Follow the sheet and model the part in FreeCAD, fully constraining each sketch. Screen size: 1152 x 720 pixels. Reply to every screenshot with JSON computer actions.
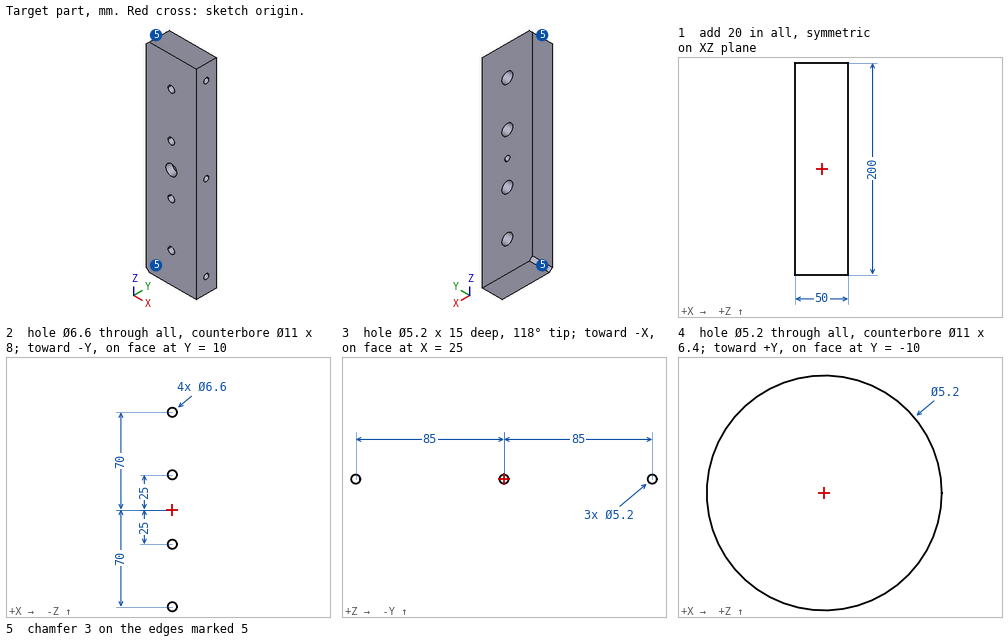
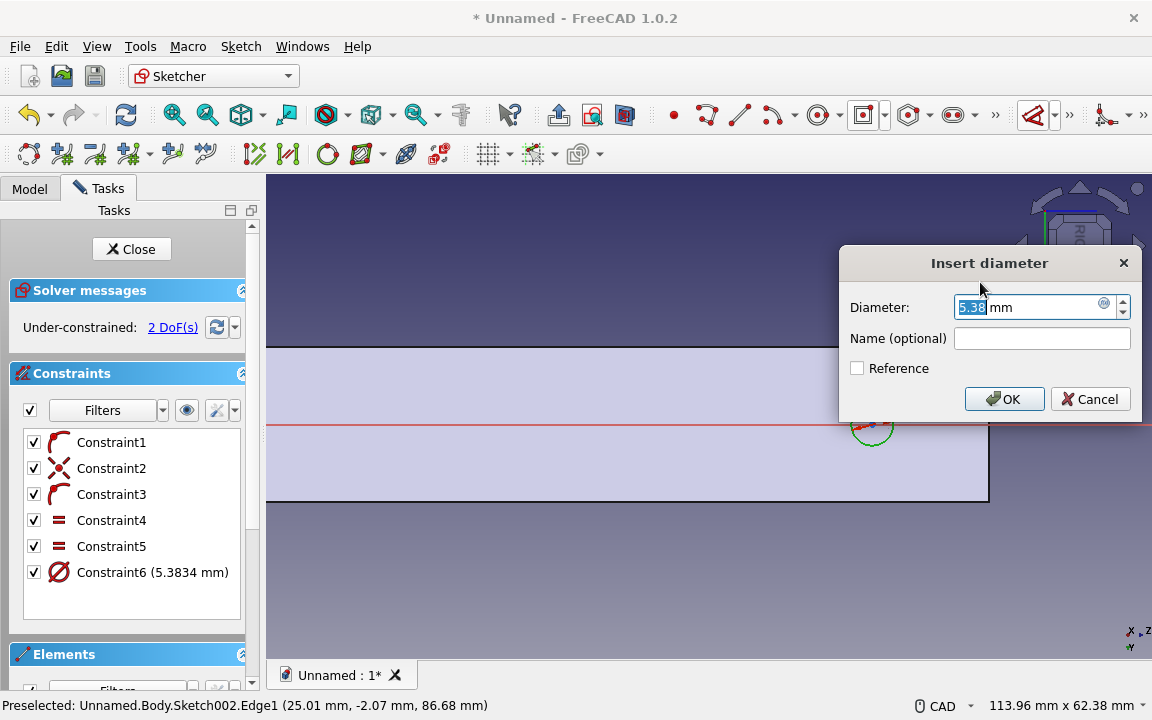
{"action": "type", "text": "5.2"}
{"action": "key", "text": "Return"}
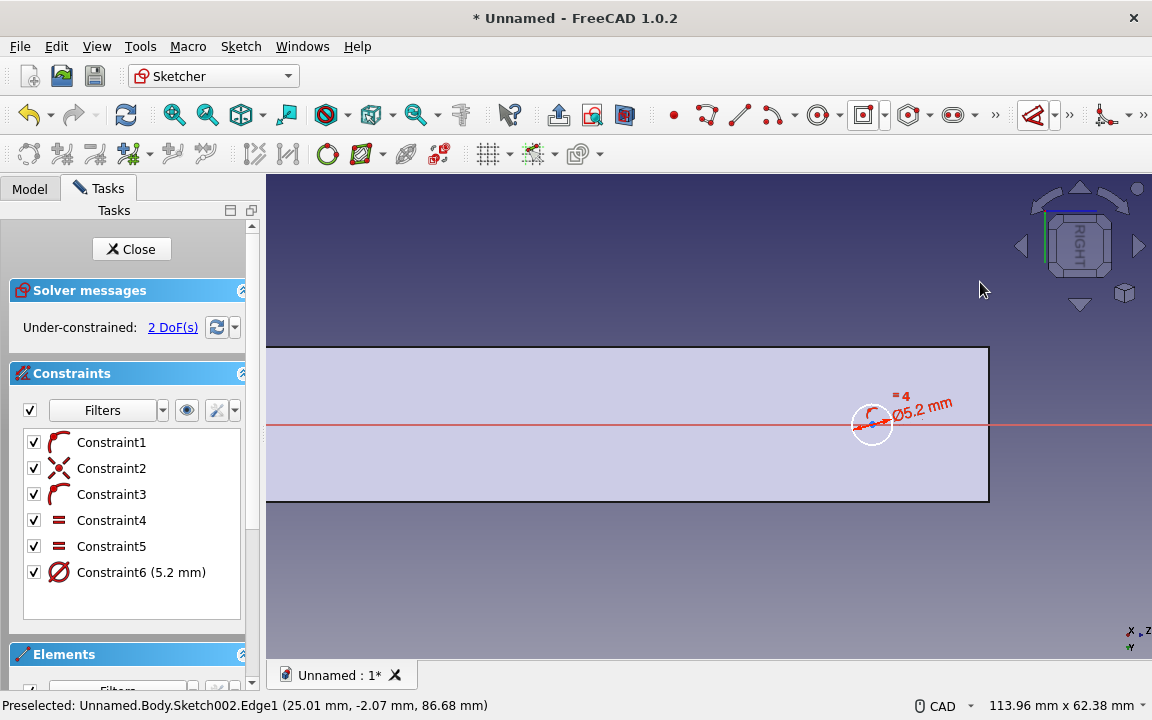
{"action": "left_click", "coordinate": [872, 425]}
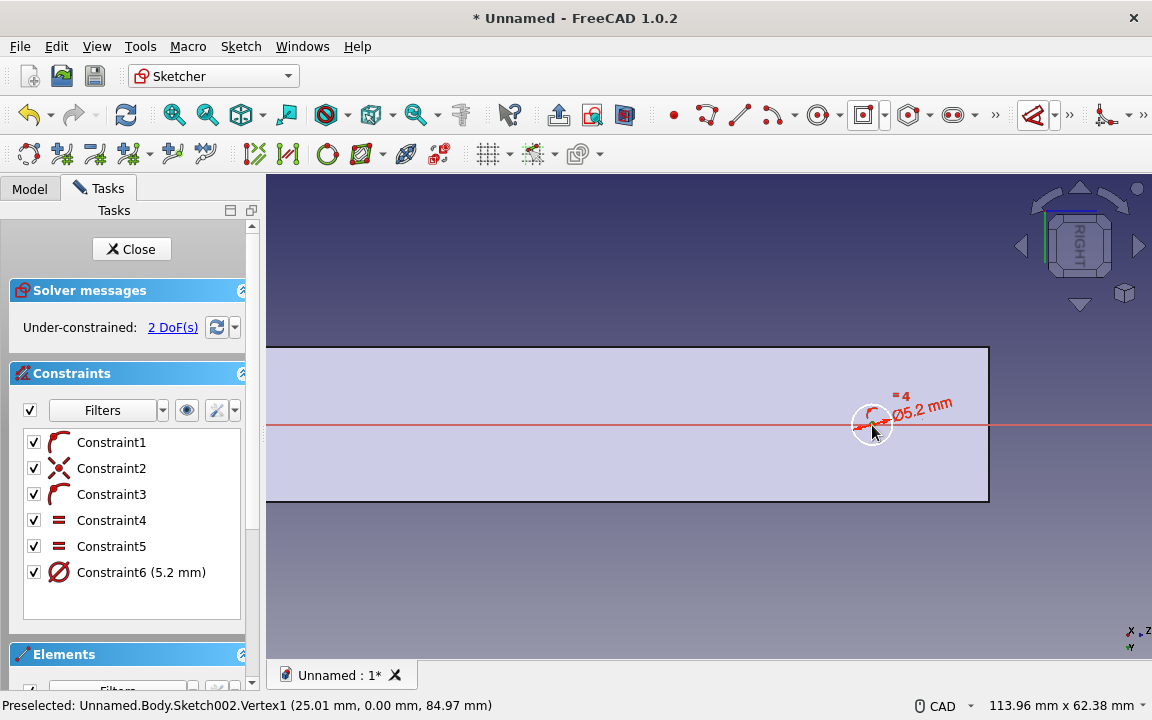
{"action": "key", "text": "l"}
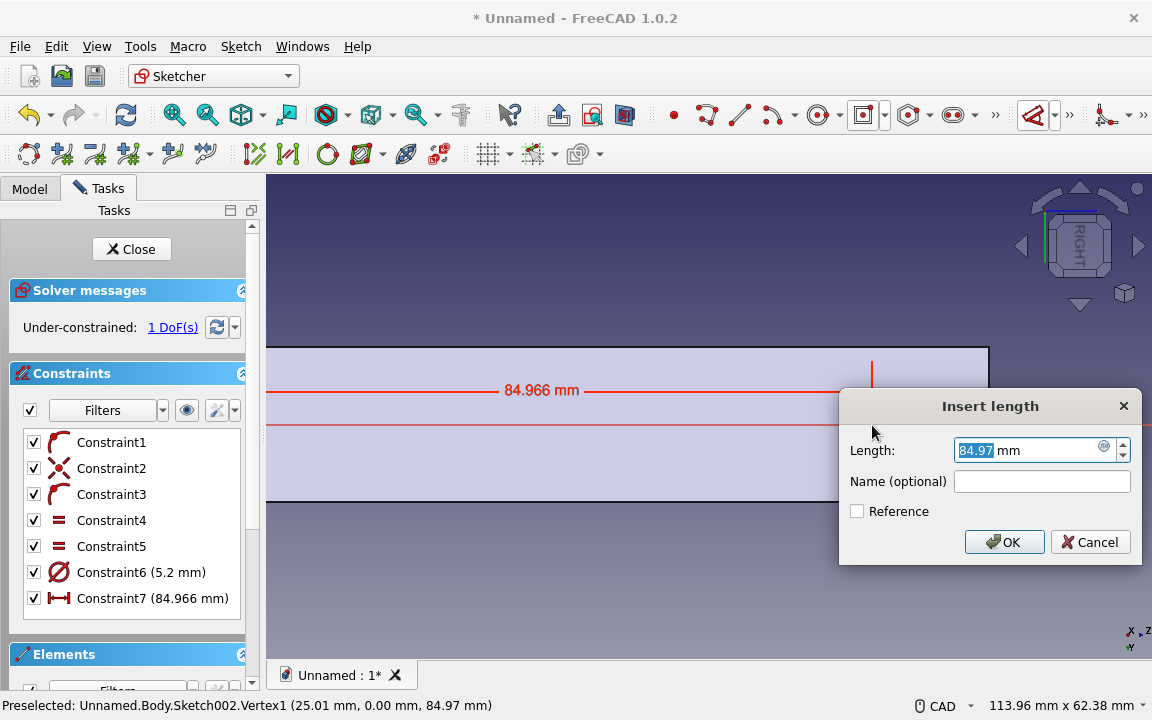
{"action": "type", "text": "85"}
{"action": "key", "text": "Return"}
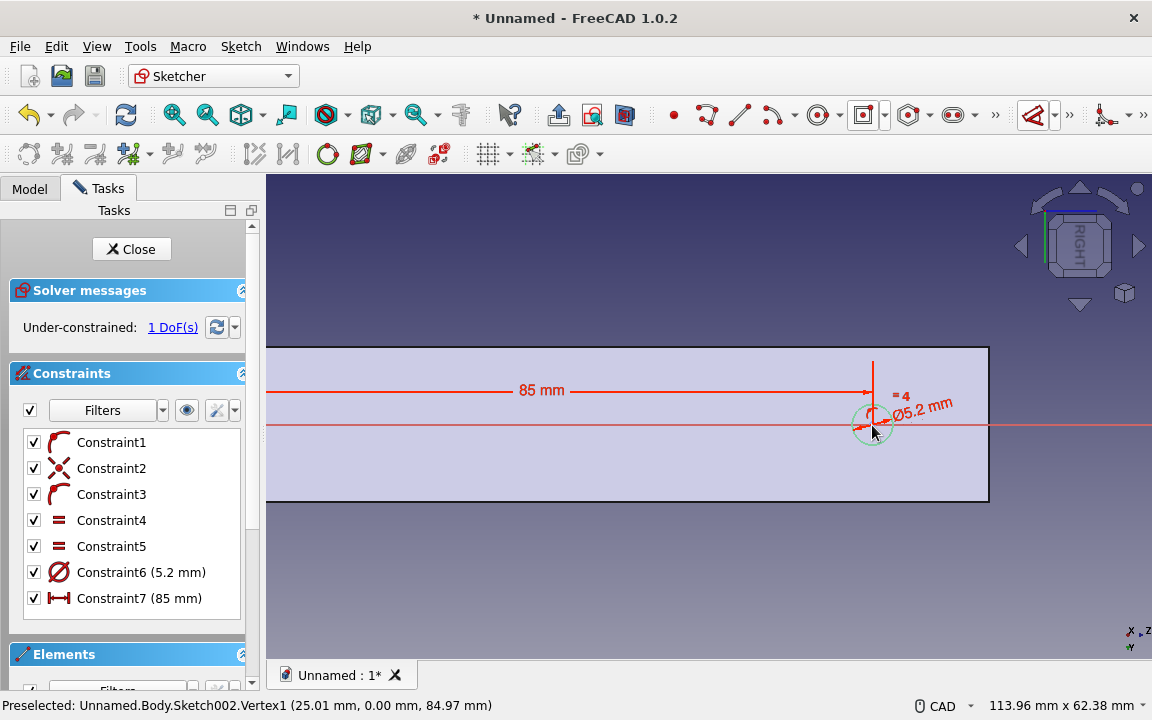
{"action": "scroll", "coordinate": [890, 412], "scroll_direction": "down", "scroll_amount": 5}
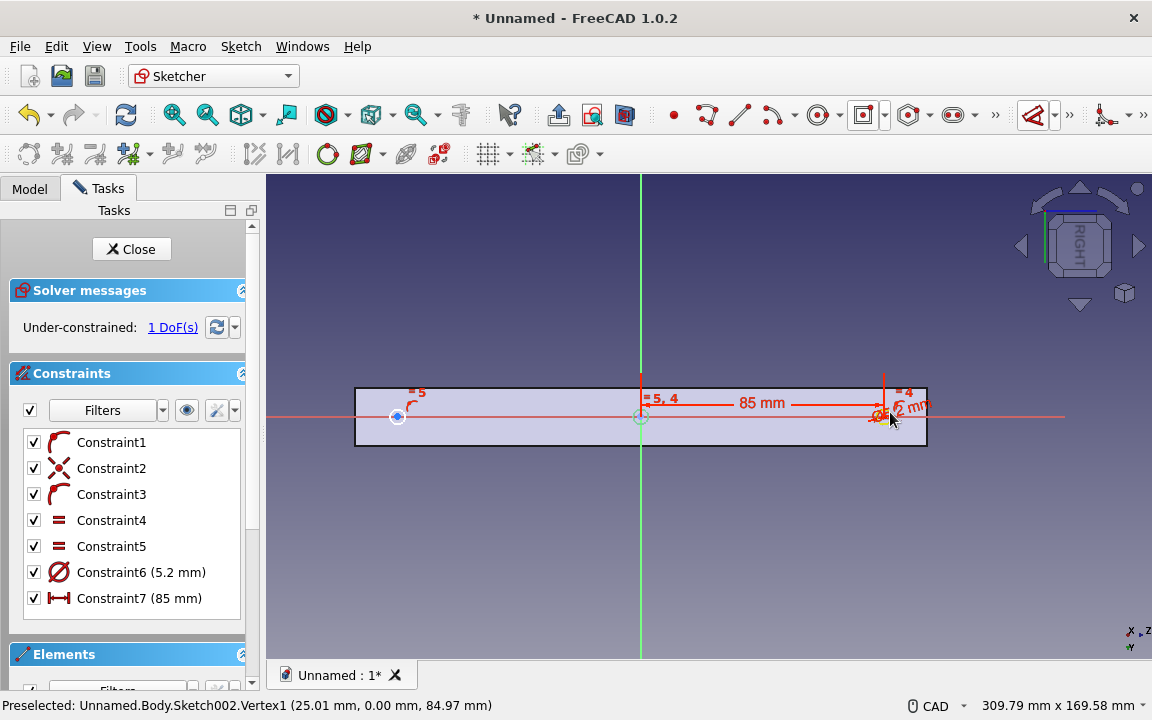
{"action": "left_click", "coordinate": [398, 417]}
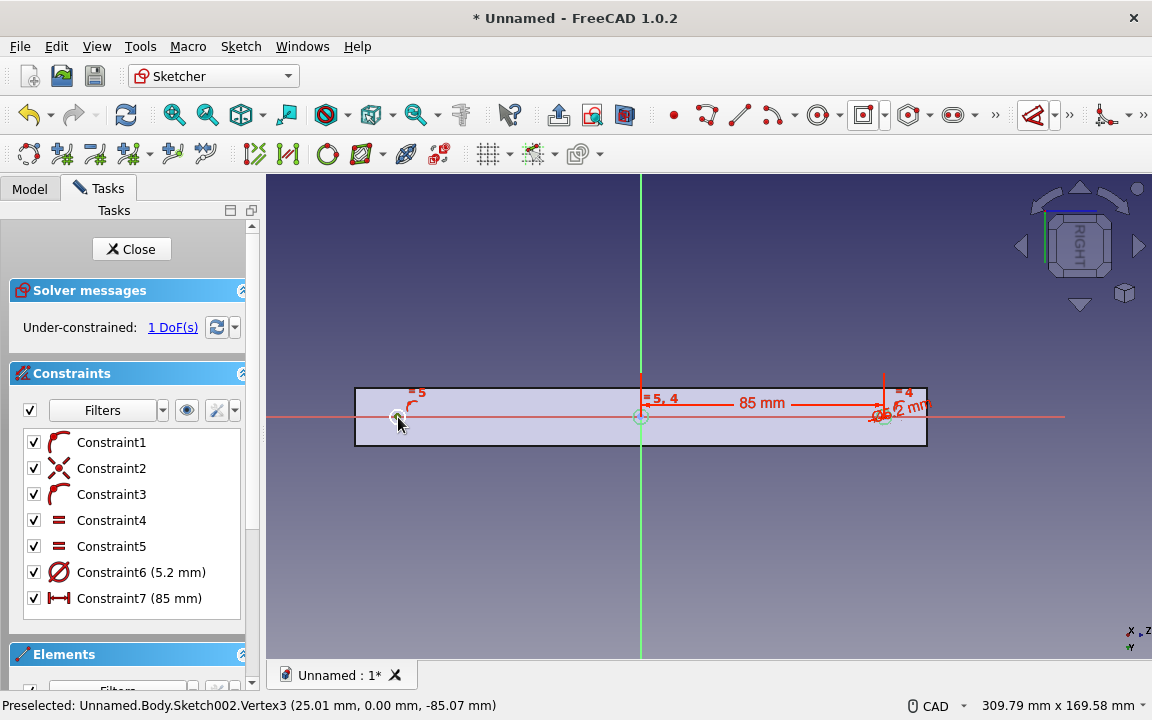
{"action": "key", "text": "l"}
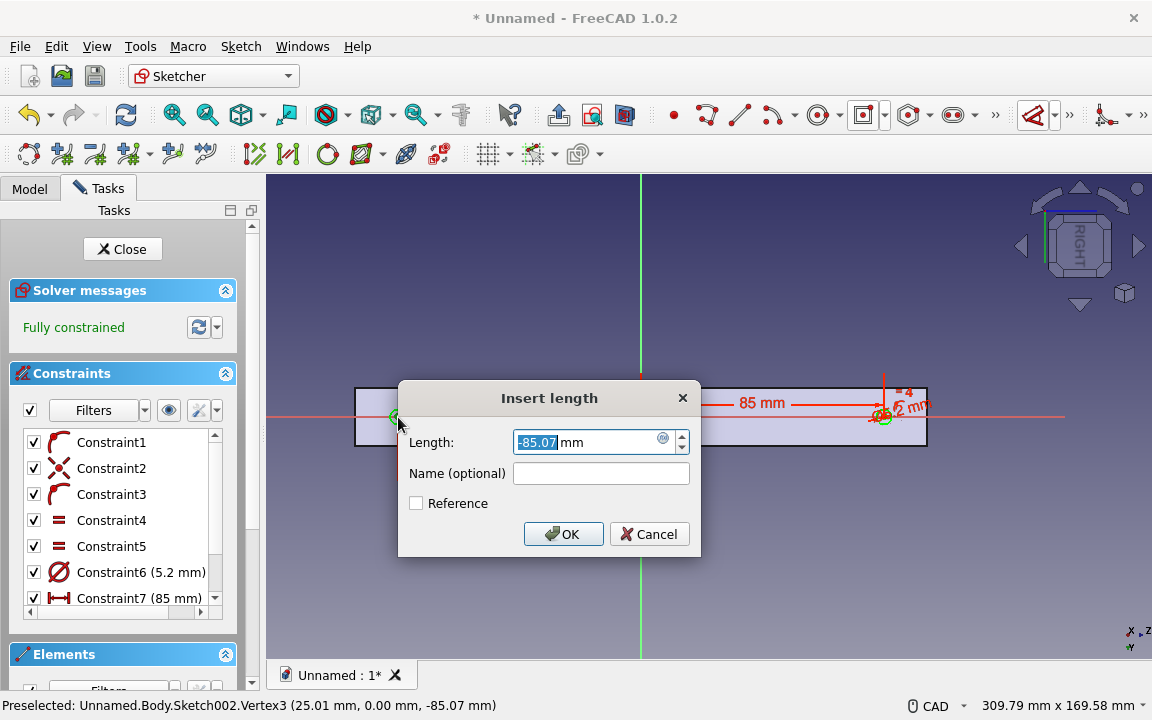
{"action": "type", "text": "-85"}
{"action": "key", "text": "Return"}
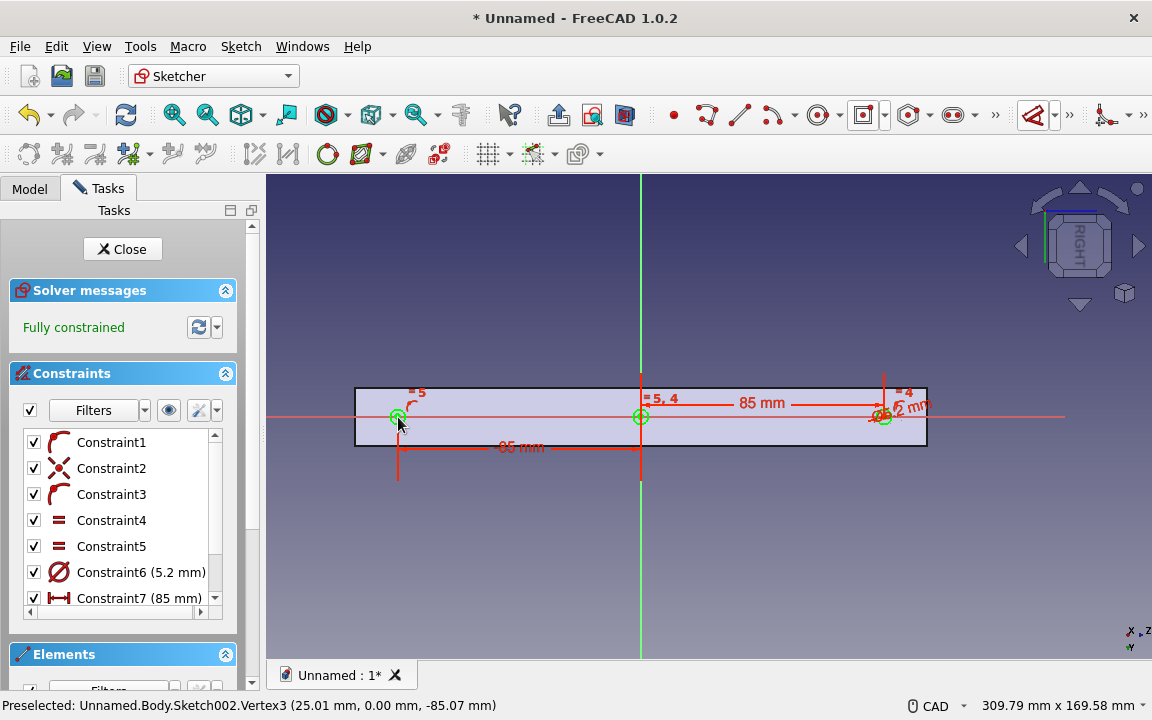
{"action": "left_click", "coordinate": [123, 249]}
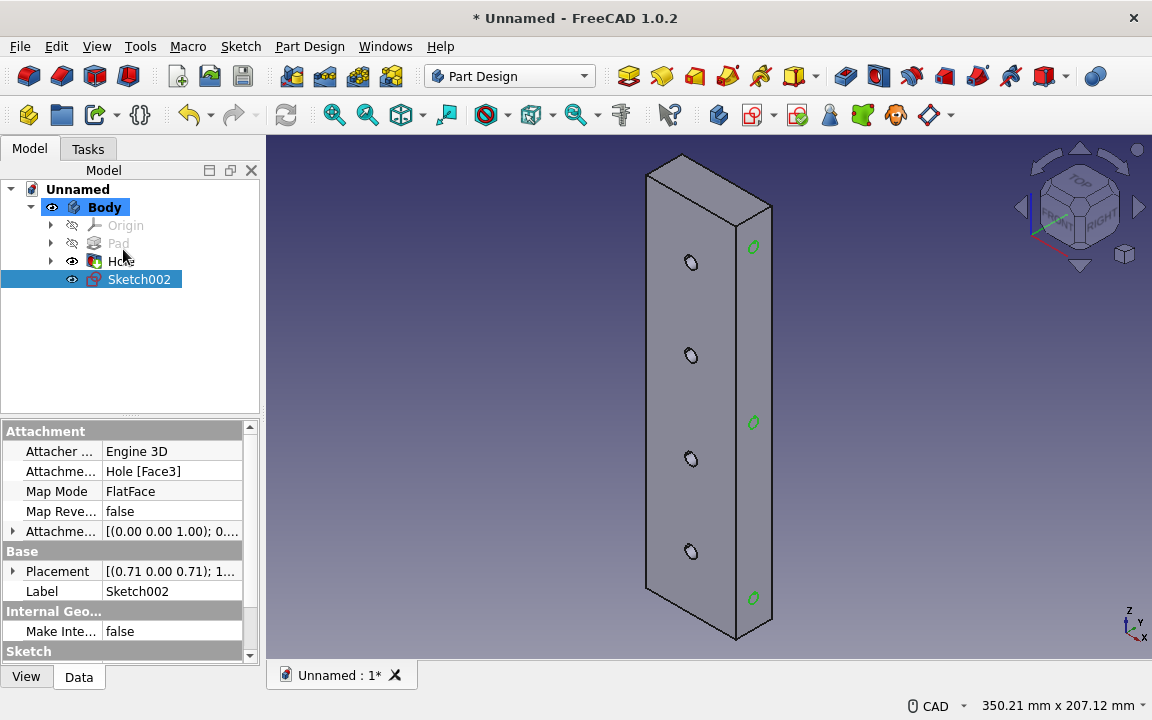
{"action": "left_click", "coordinate": [879, 76]}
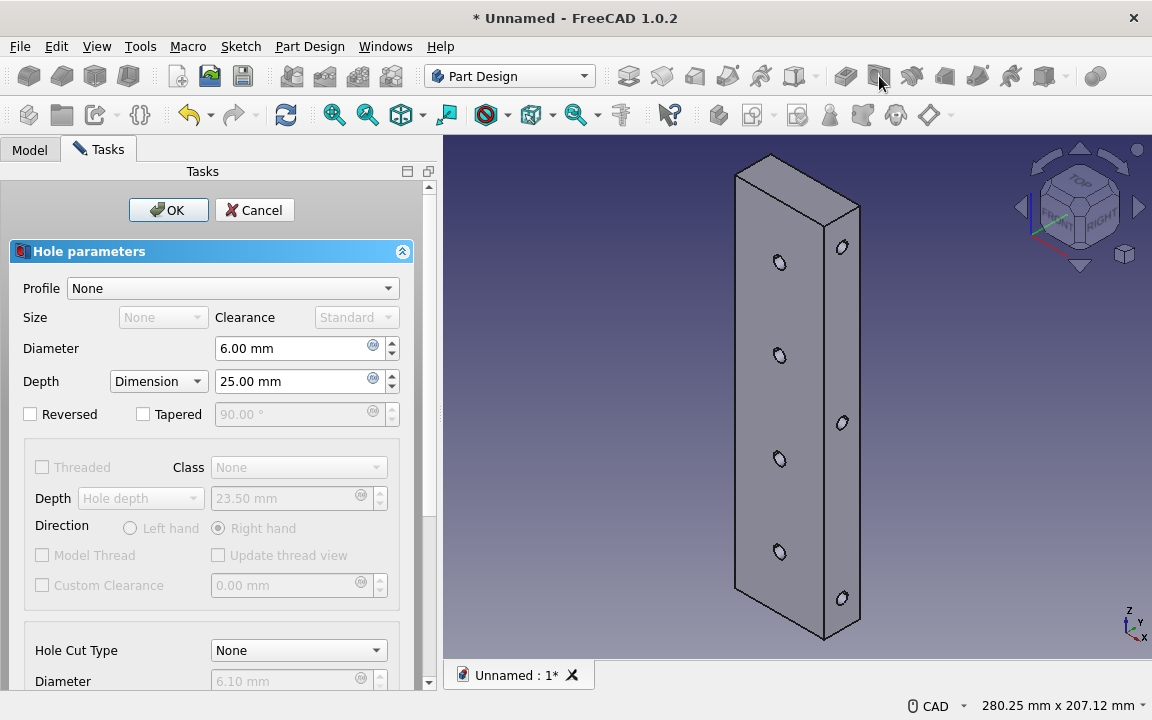
{"action": "triple_click", "coordinate": [300, 348]}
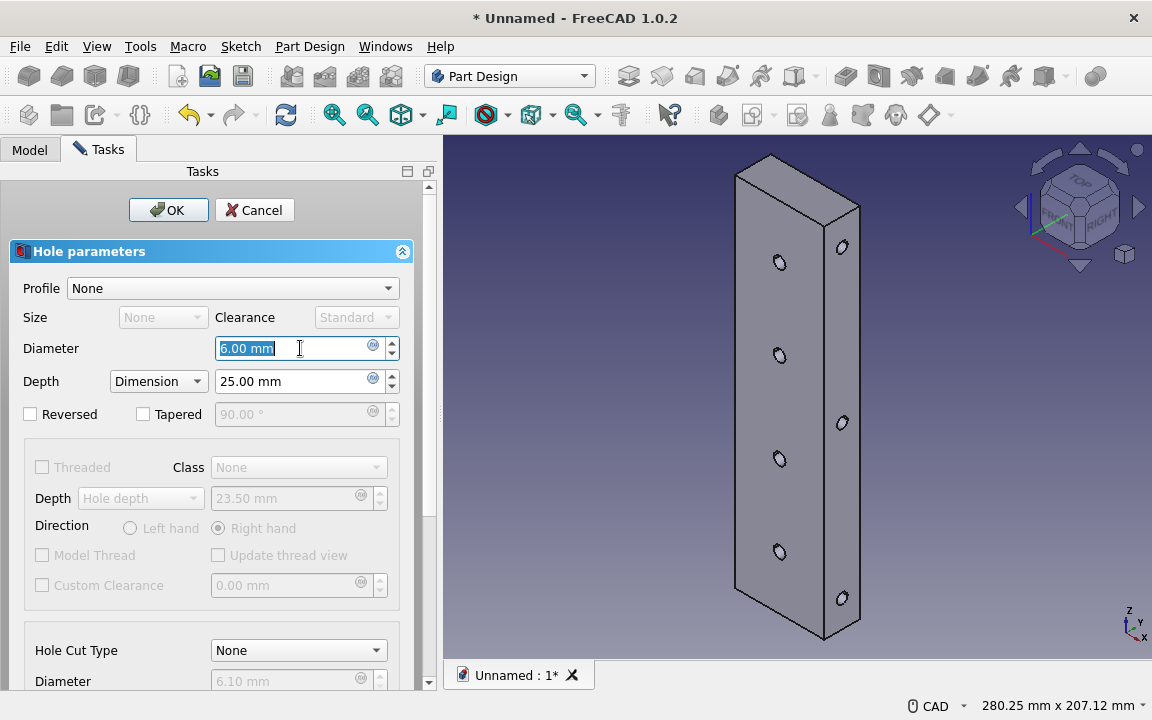
{"action": "type", "text": "5.2"}
{"action": "key", "text": "Tab"}